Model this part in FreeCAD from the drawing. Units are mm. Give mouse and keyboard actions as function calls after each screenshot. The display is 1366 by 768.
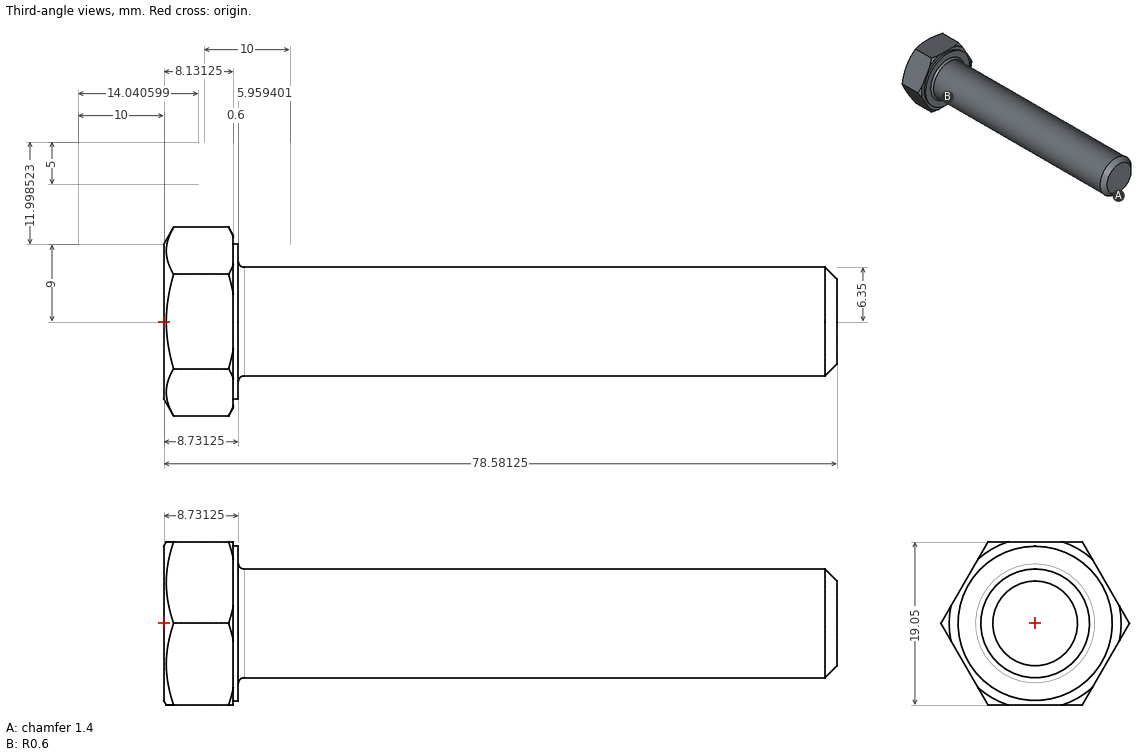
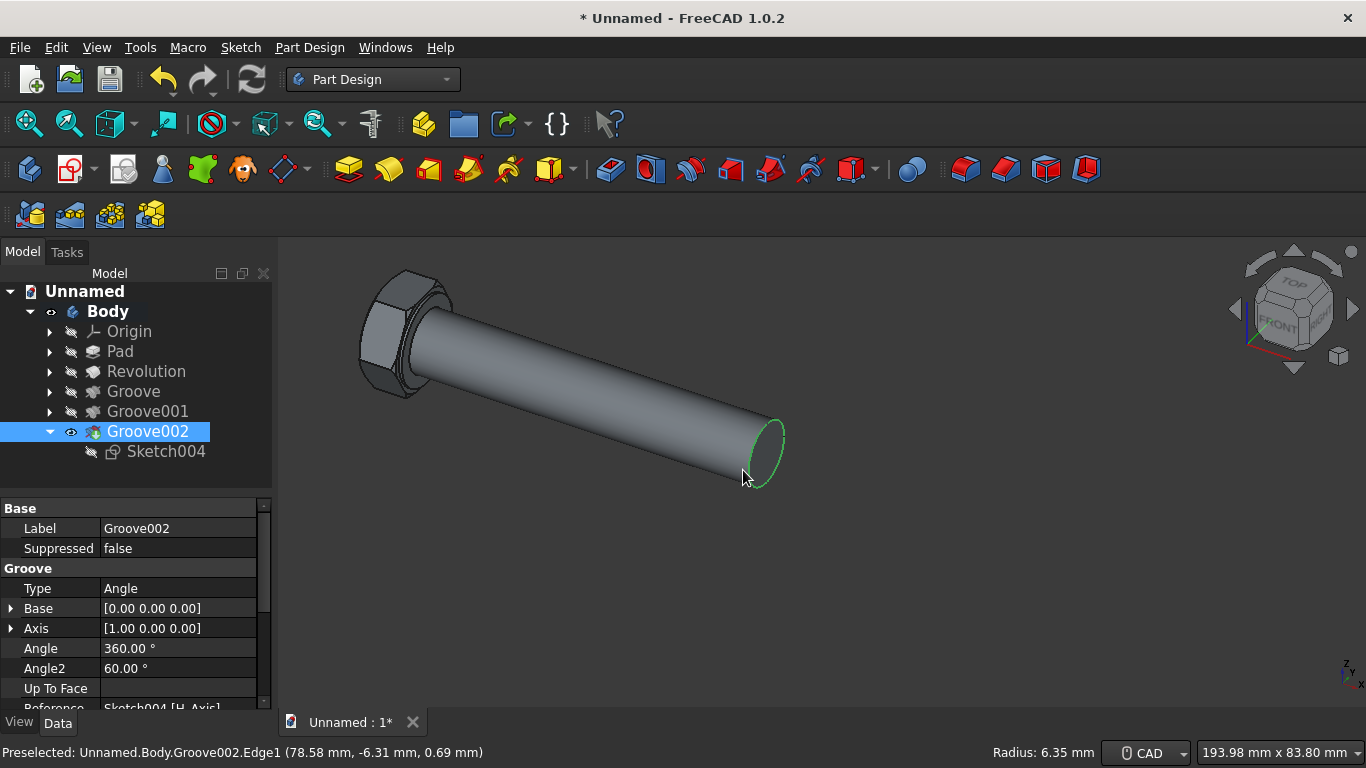
click(1006, 170)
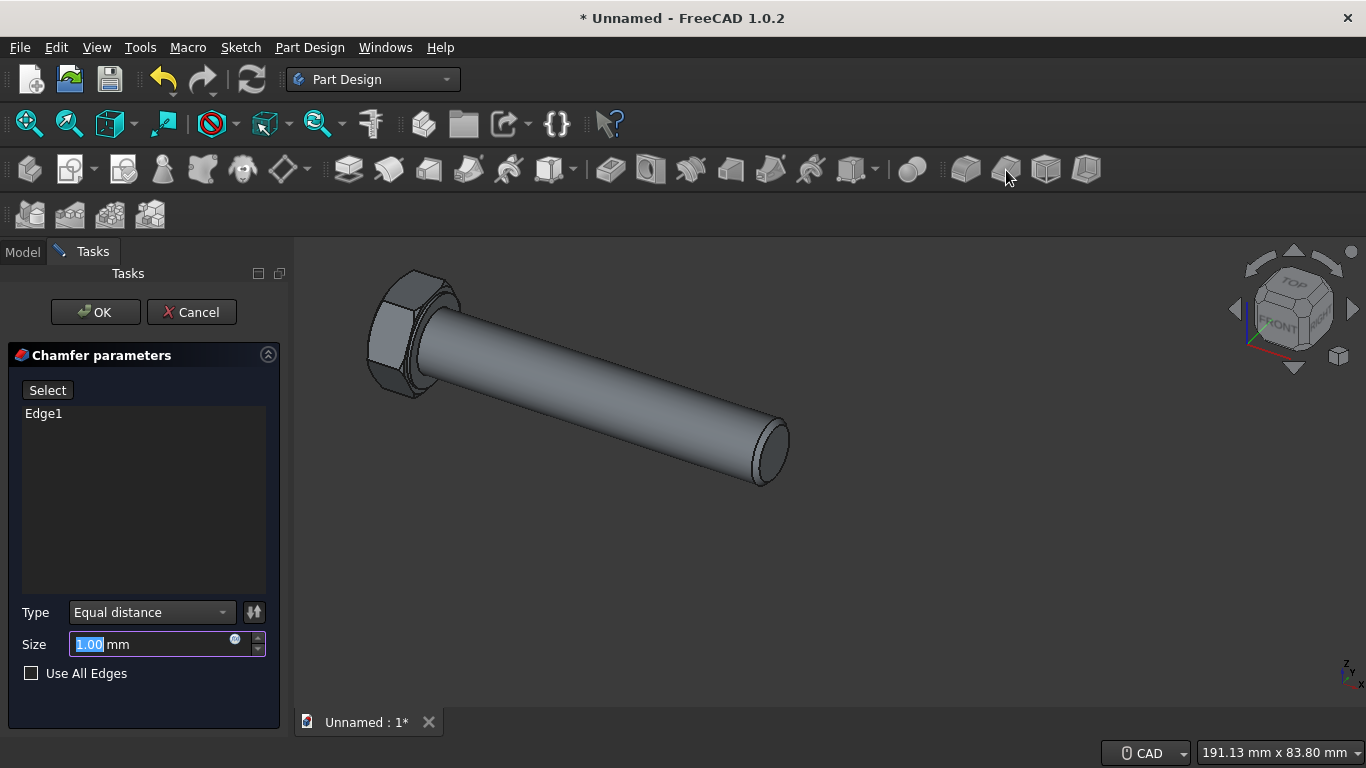
text(1.4)
key(Tab)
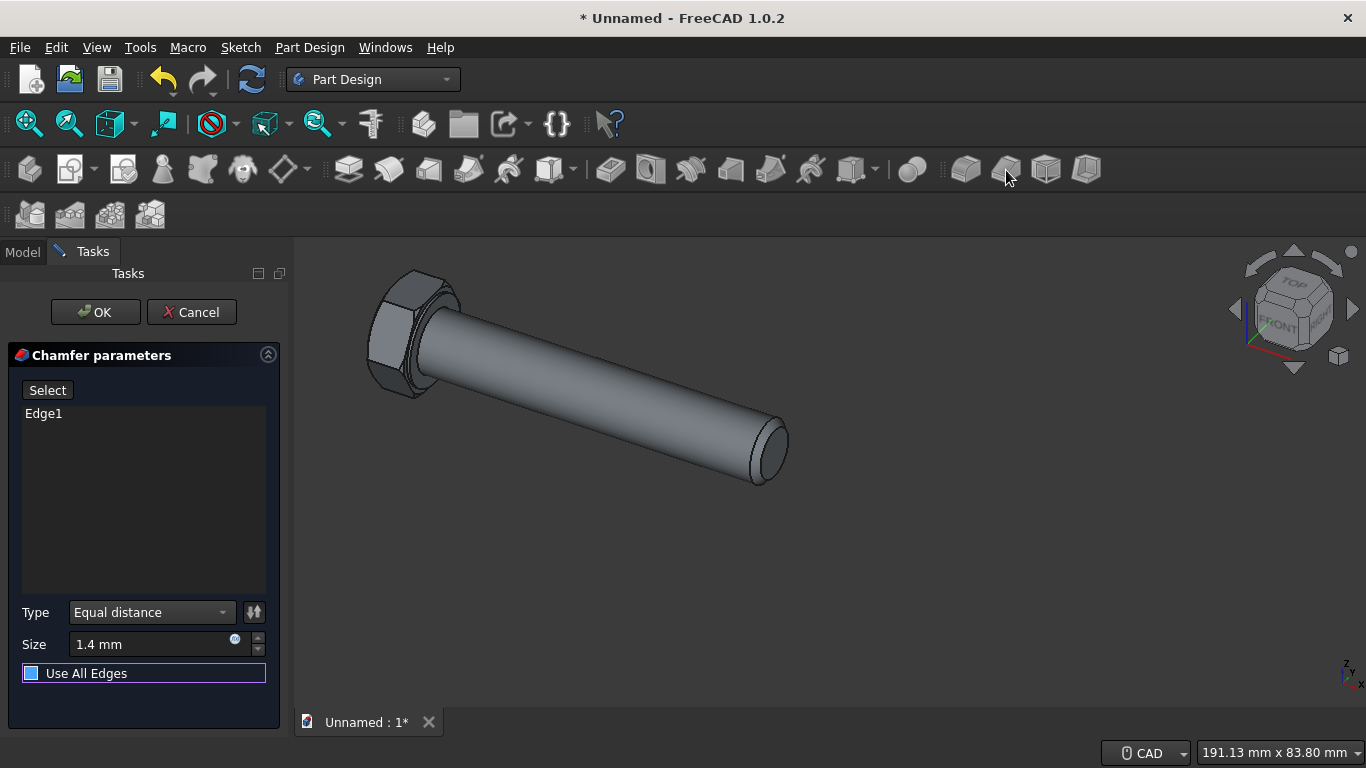
click(96, 312)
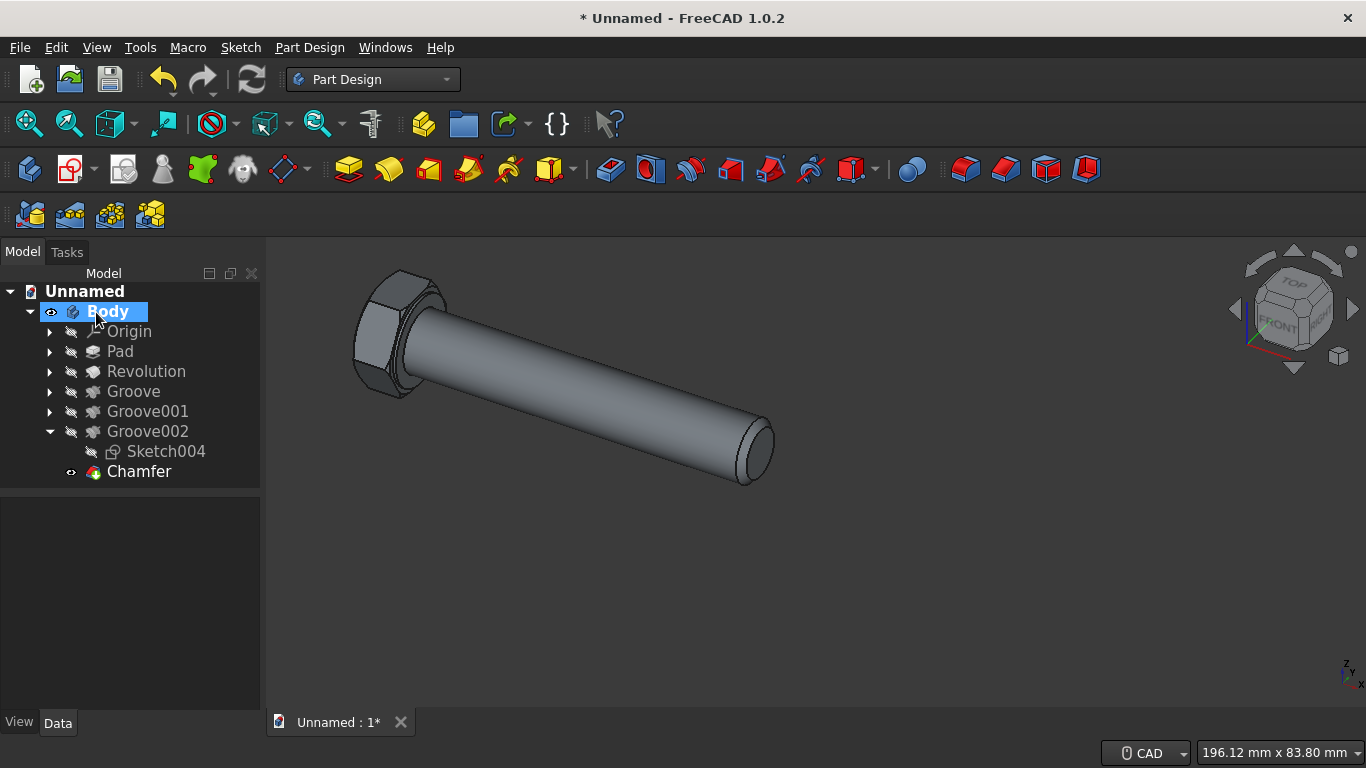
key(0)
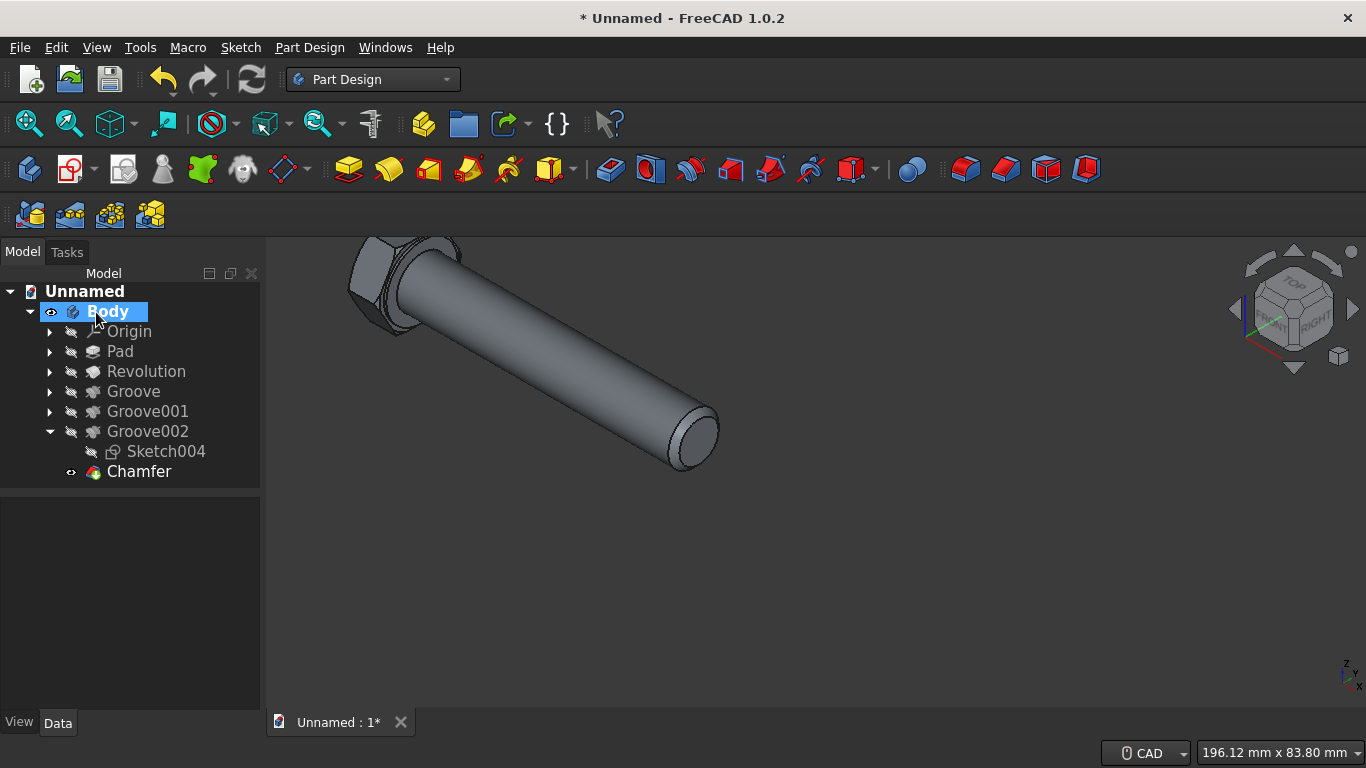
click(30, 124)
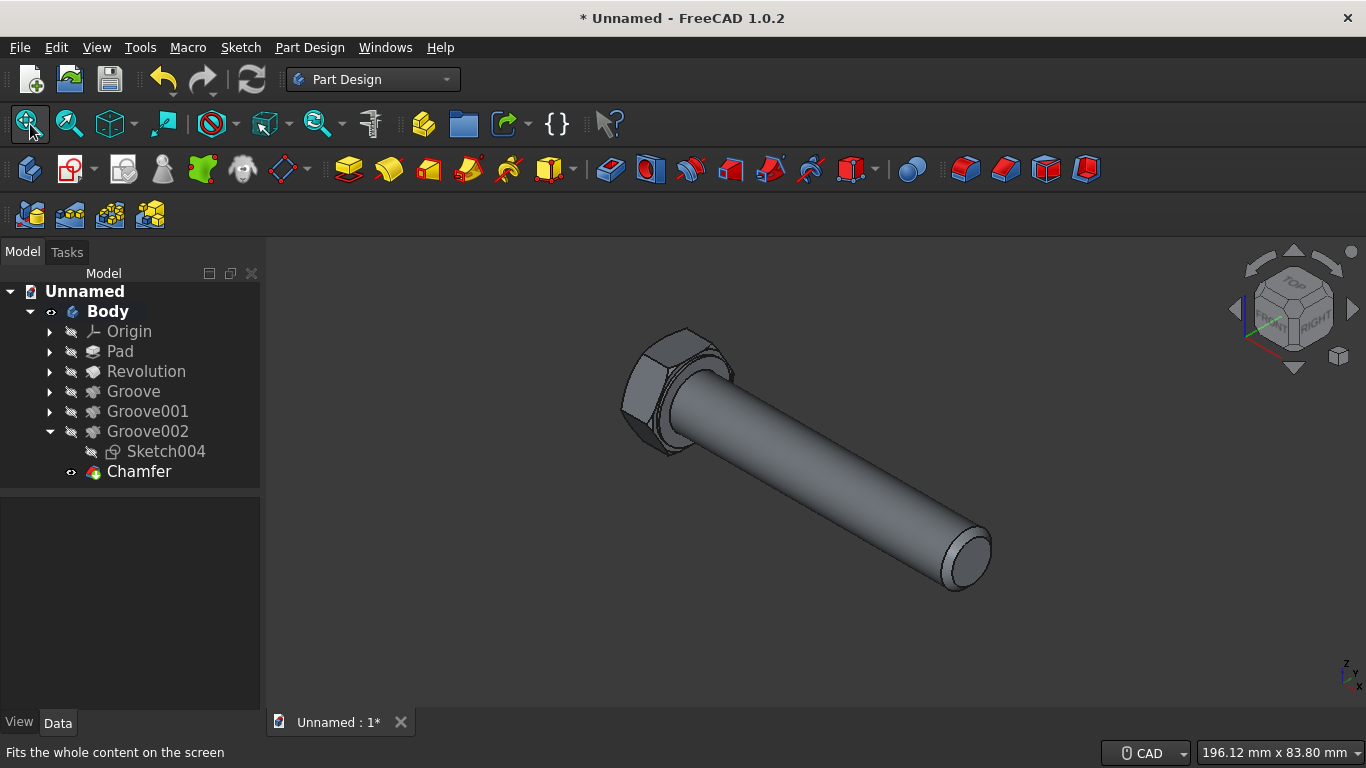
key(2)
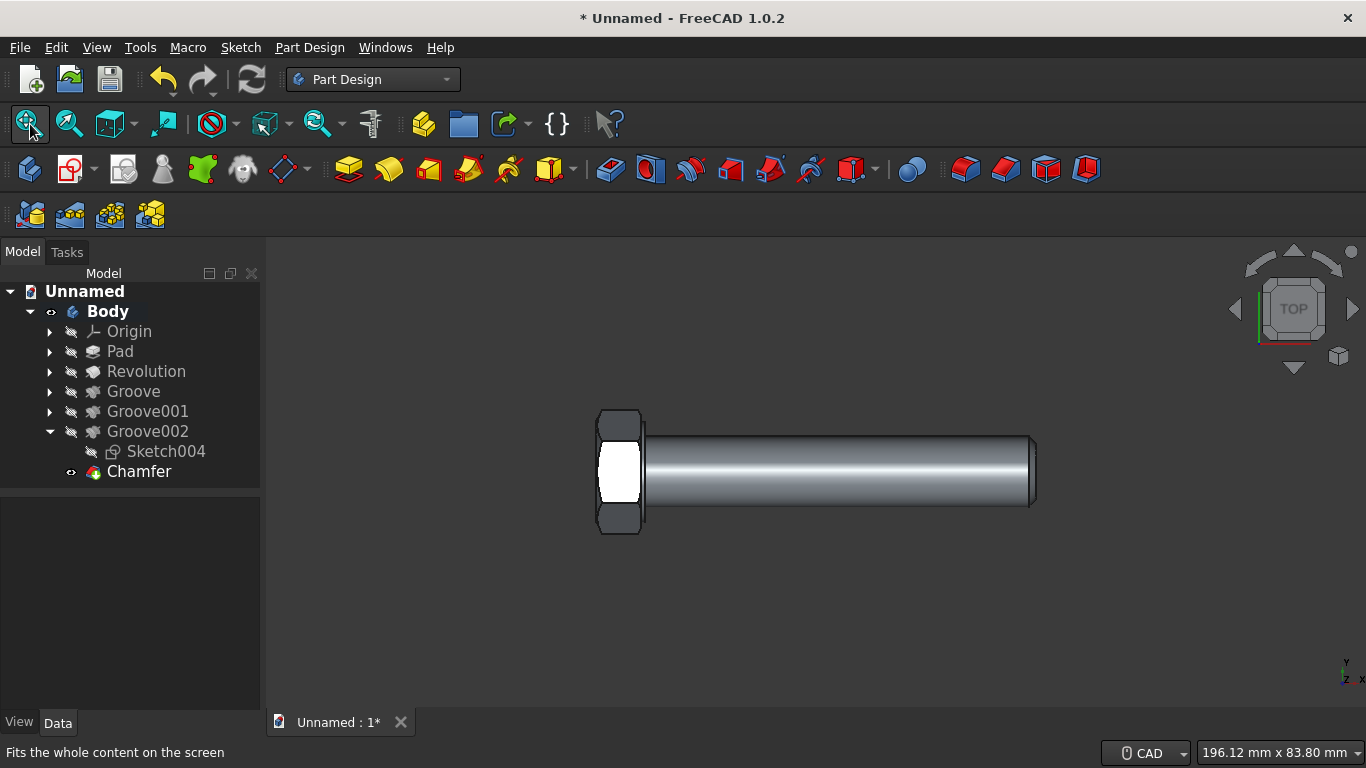
click(30, 124)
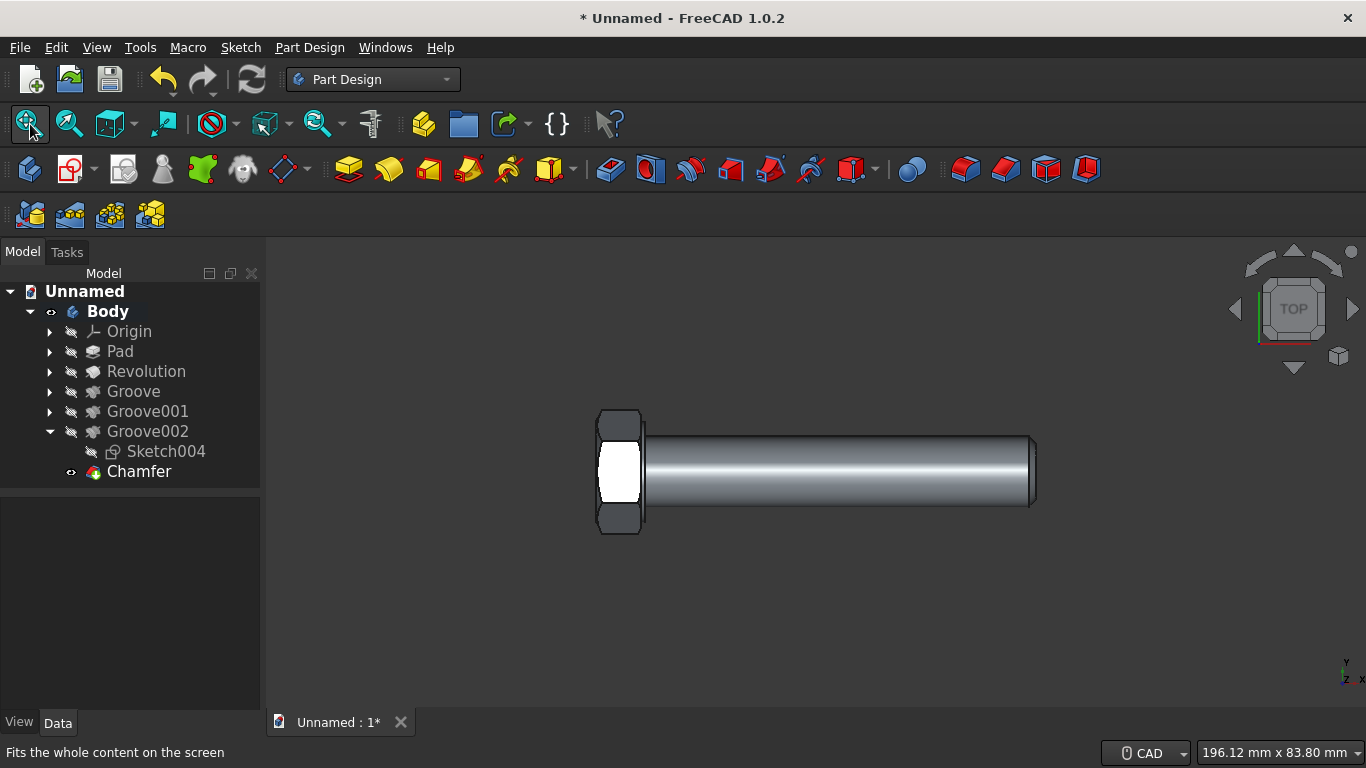
key(1)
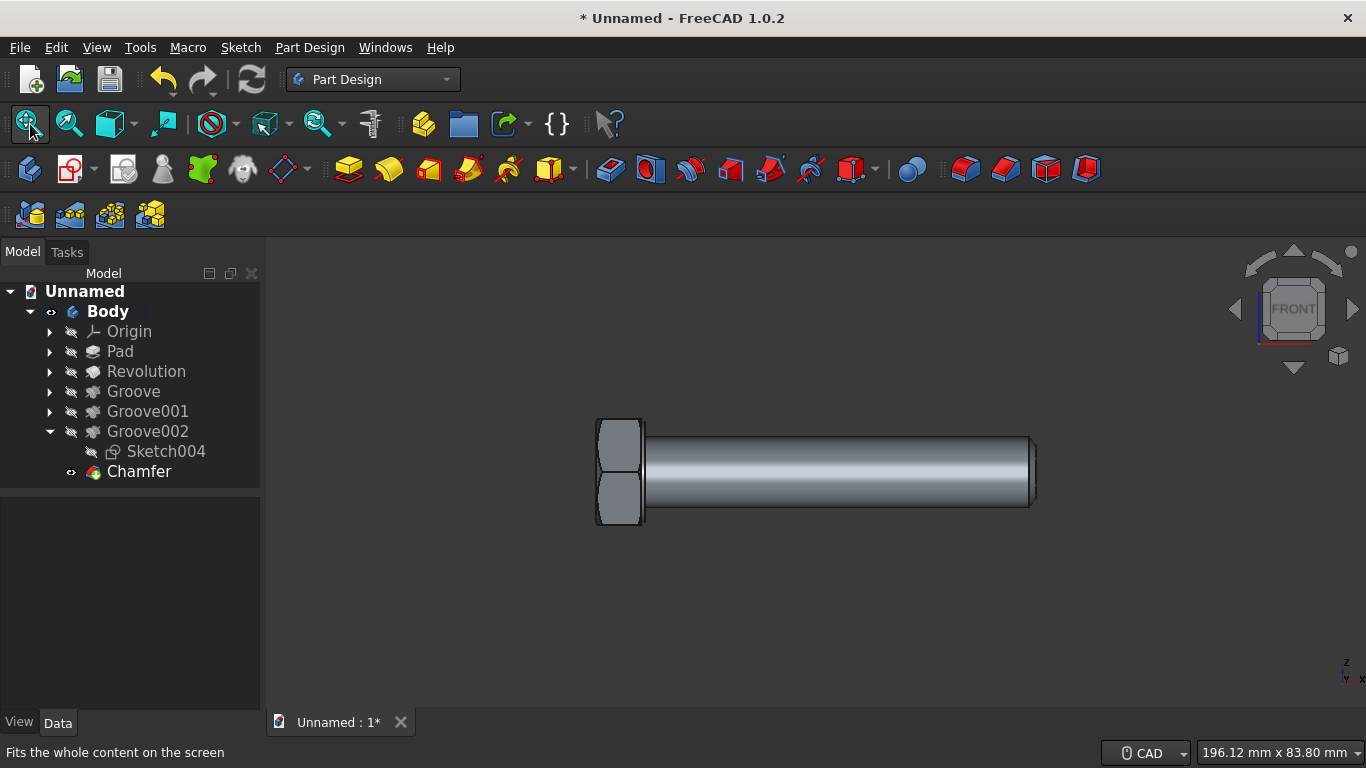
click(30, 124)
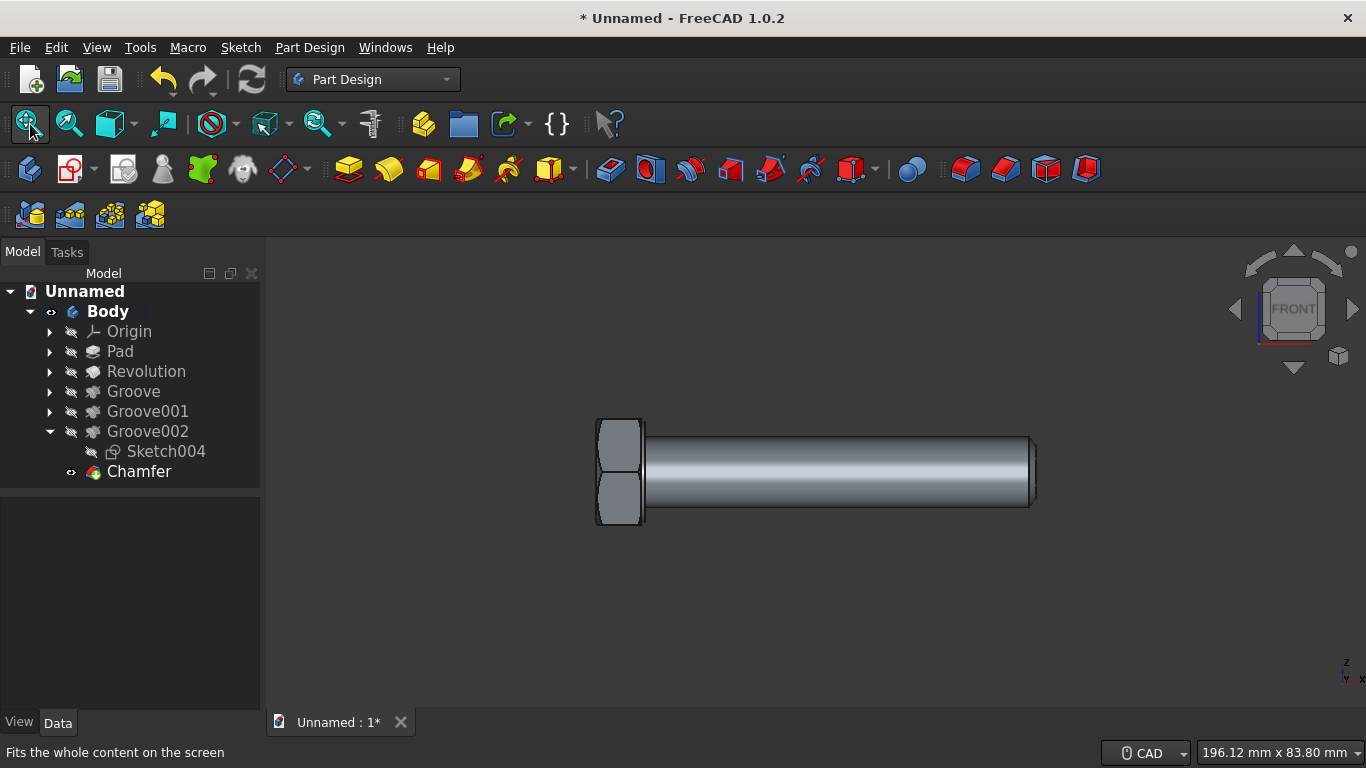
key(3)